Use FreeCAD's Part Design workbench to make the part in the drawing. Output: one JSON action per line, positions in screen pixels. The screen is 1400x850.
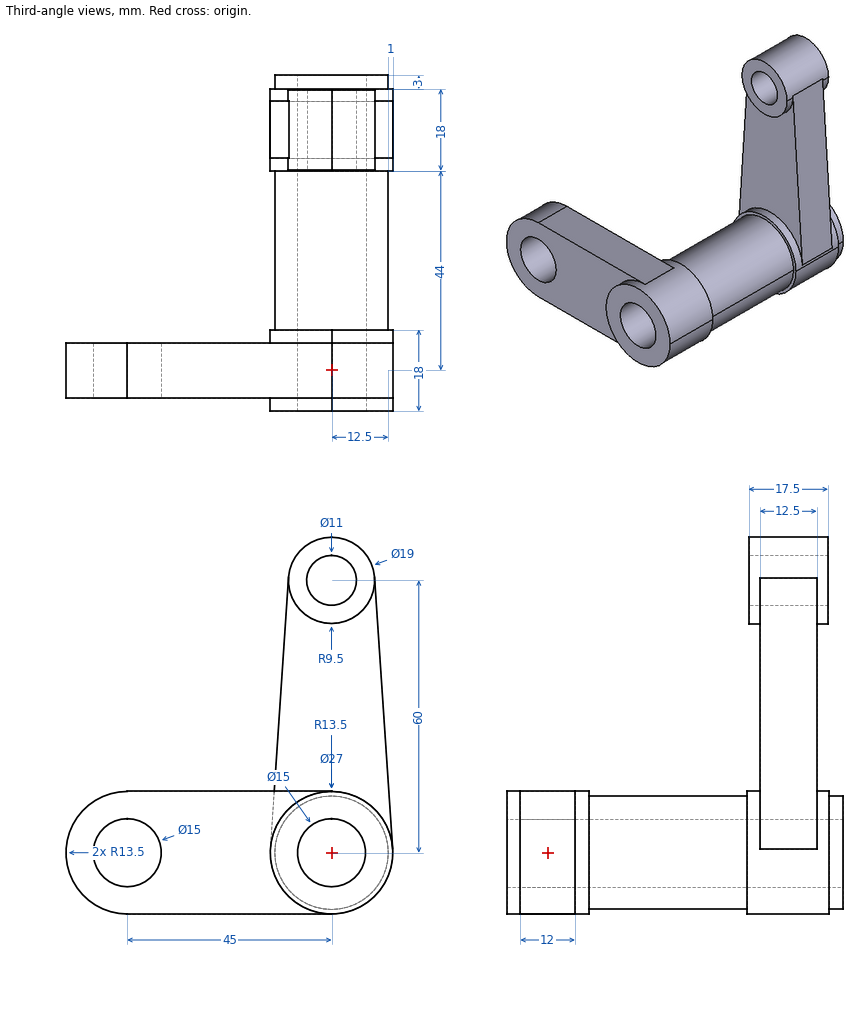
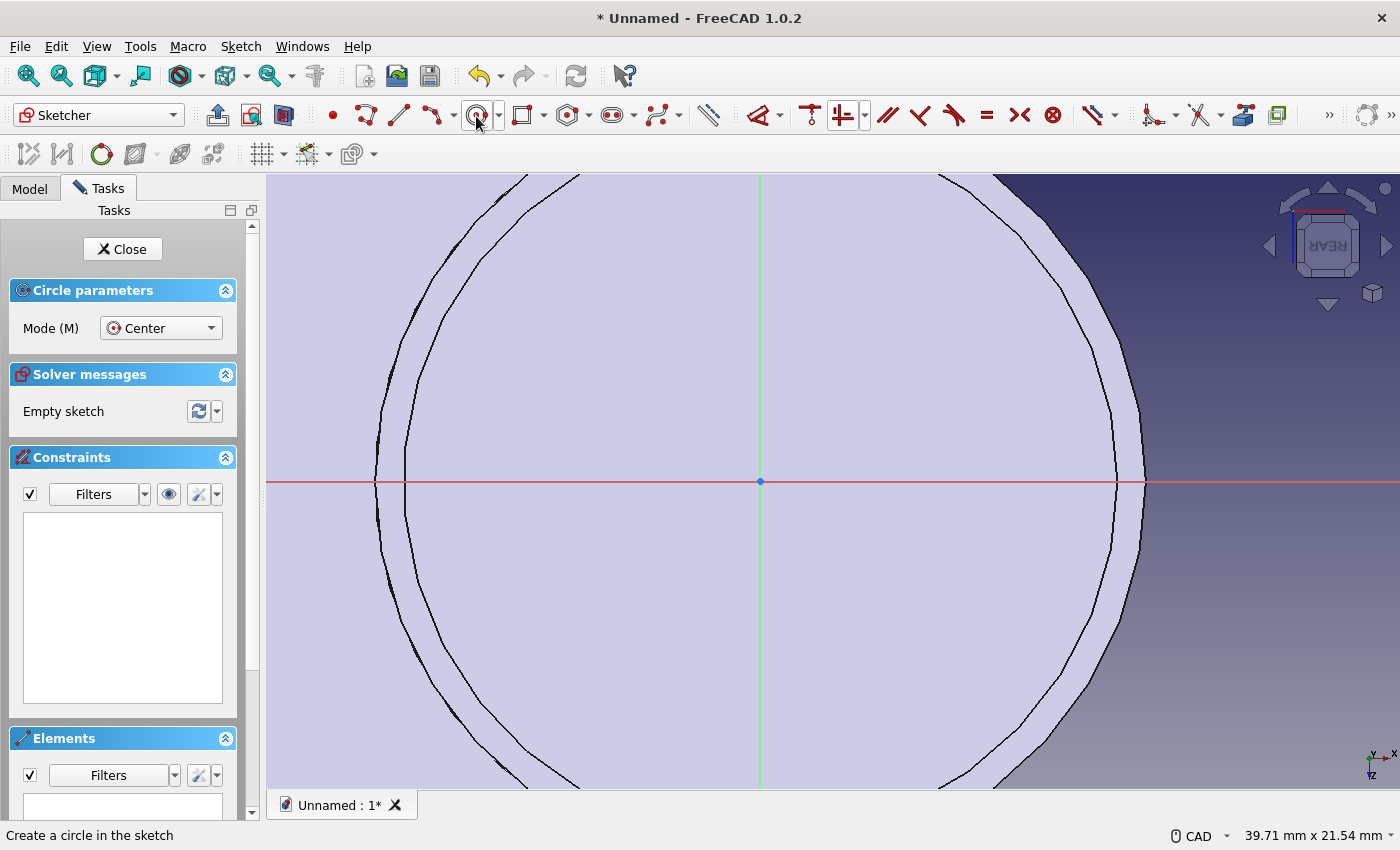
{"action": "left_click", "coordinate": [760, 481]}
{"action": "left_click", "coordinate": [912, 330]}
{"action": "key", "text": "Escape"}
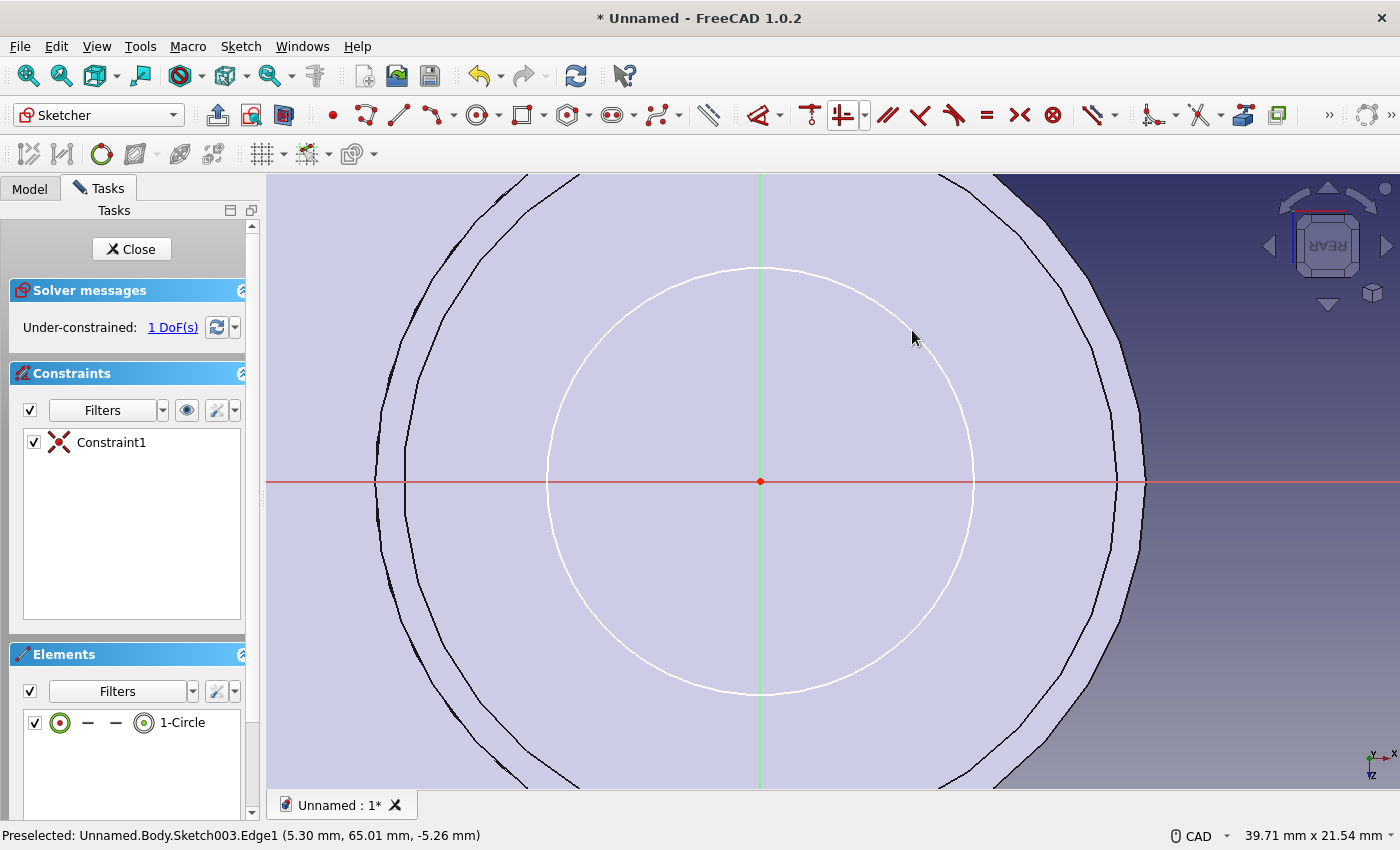
{"action": "left_click", "coordinate": [758, 116]}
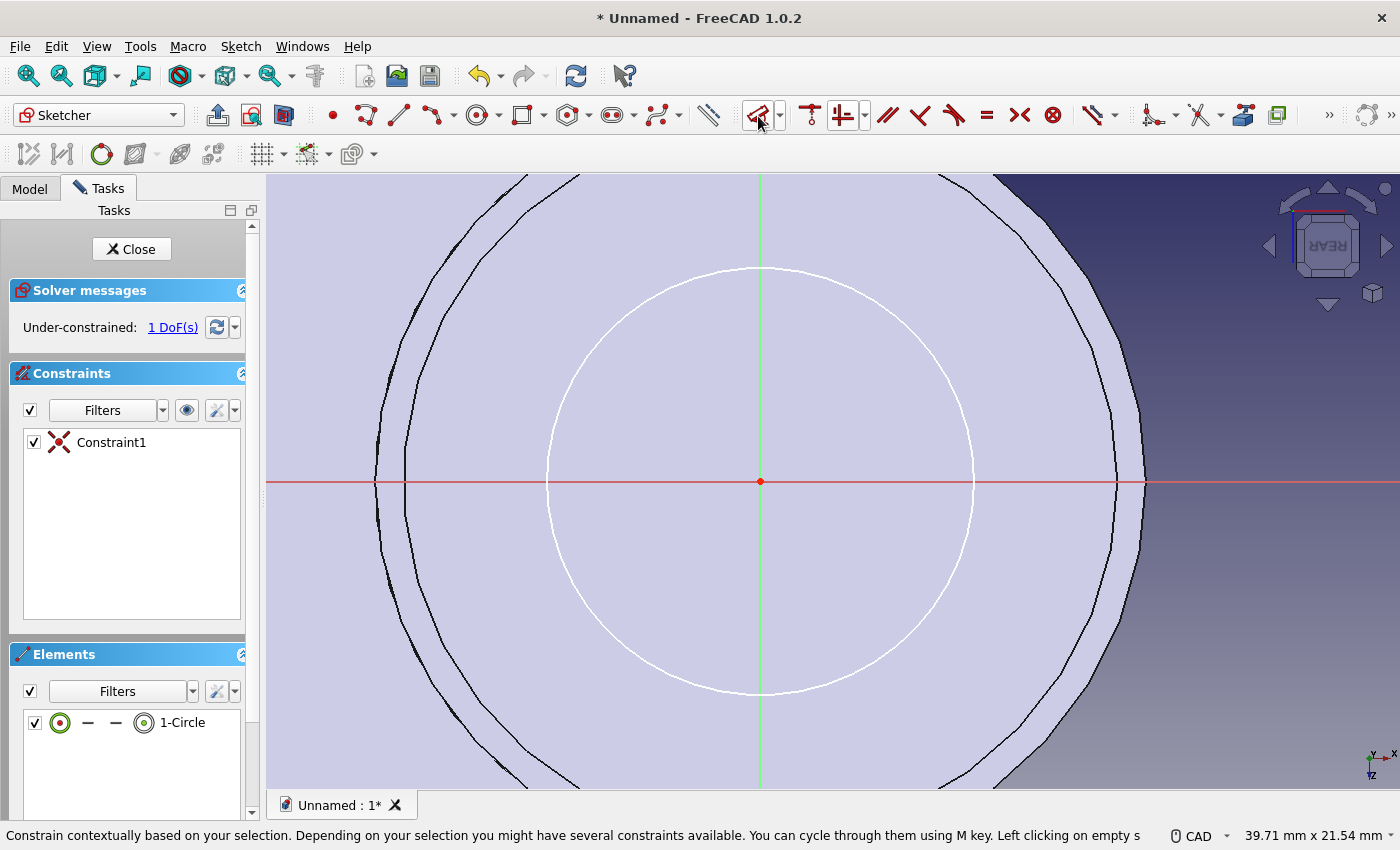
{"action": "left_click", "coordinate": [911, 330]}
{"action": "left_click", "coordinate": [934, 307]}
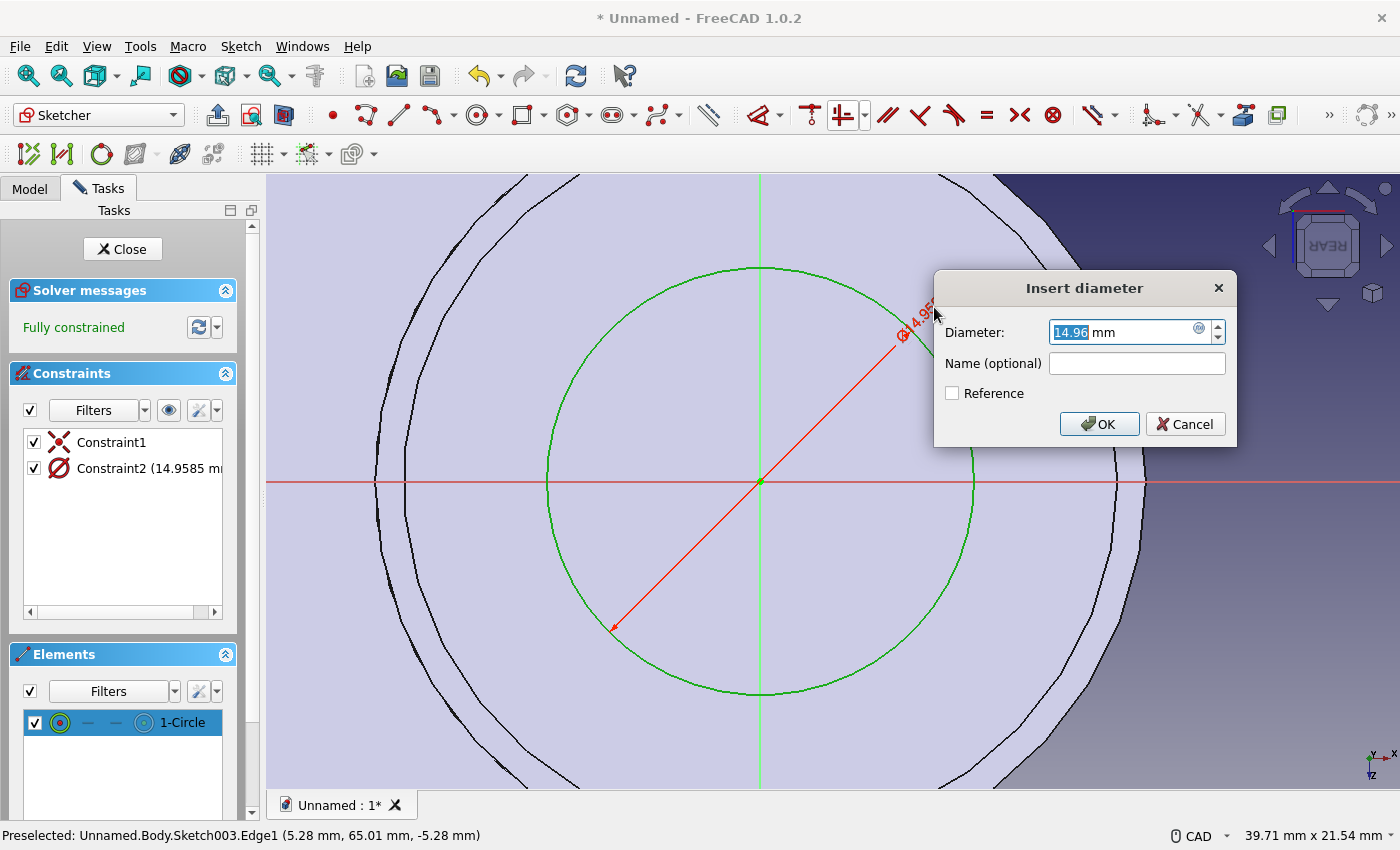
{"action": "type", "text": "15"}
{"action": "key", "text": "Return"}
{"action": "key", "text": "Escape"}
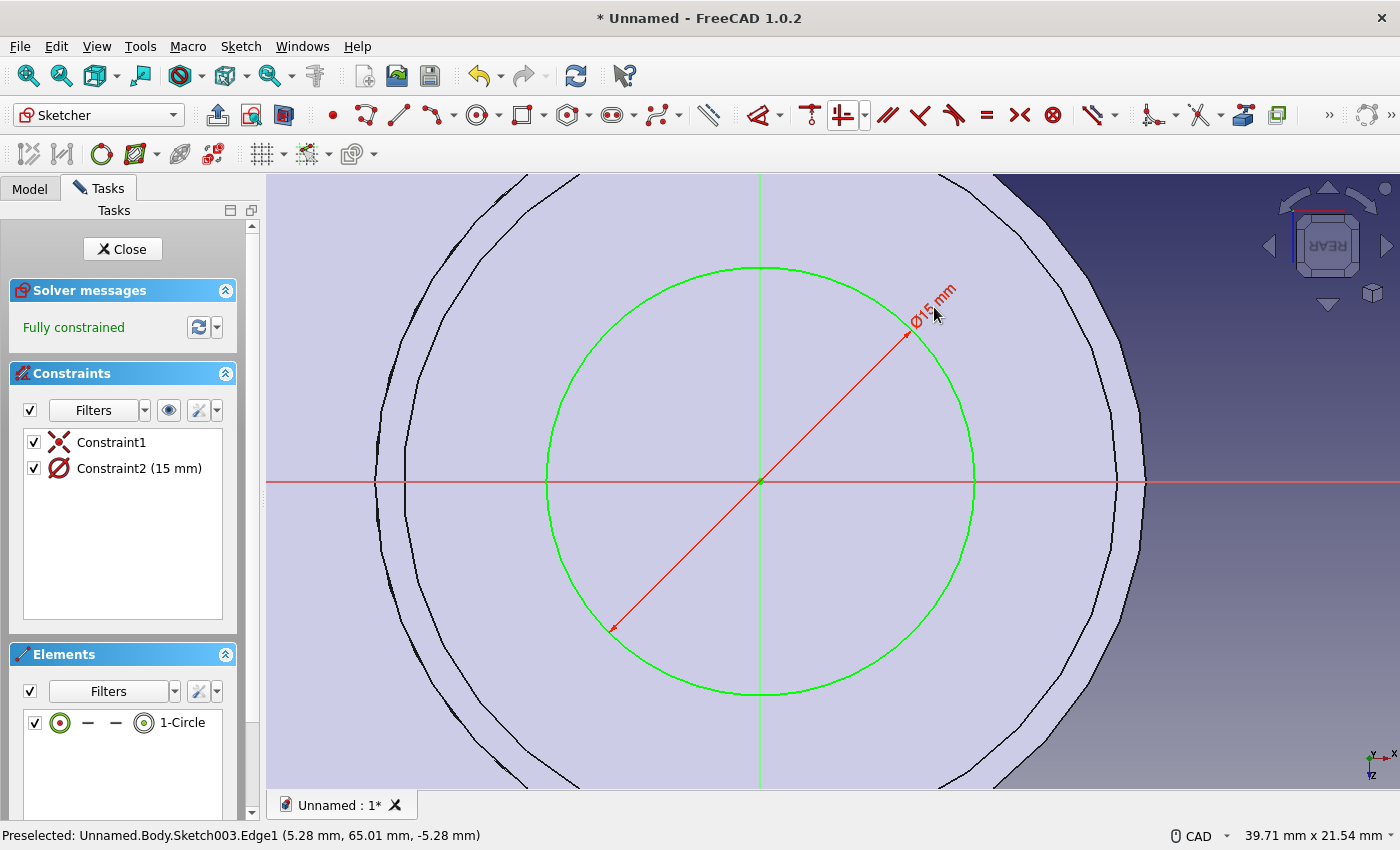
{"action": "left_click", "coordinate": [123, 249]}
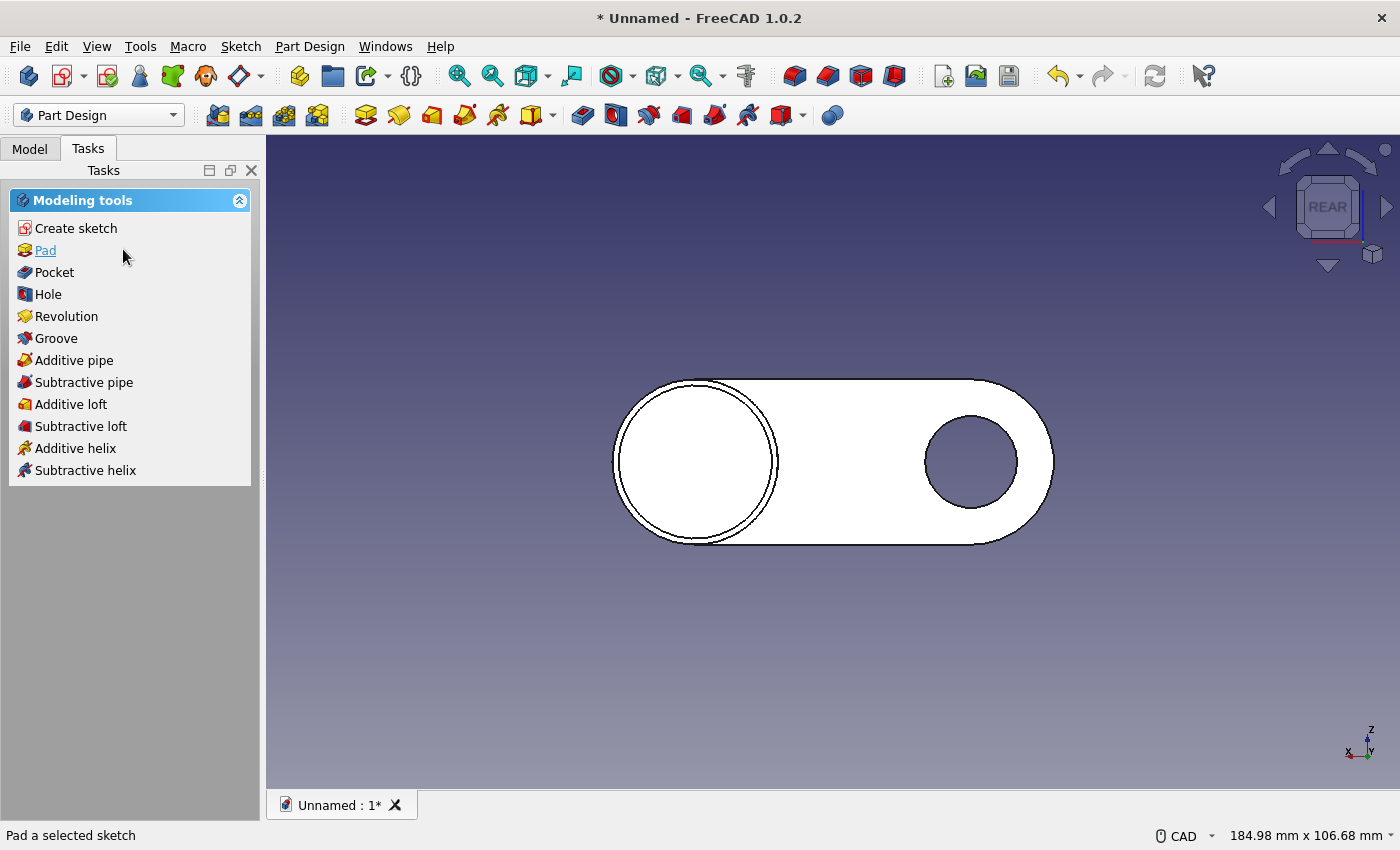
{"action": "left_click", "coordinate": [583, 116]}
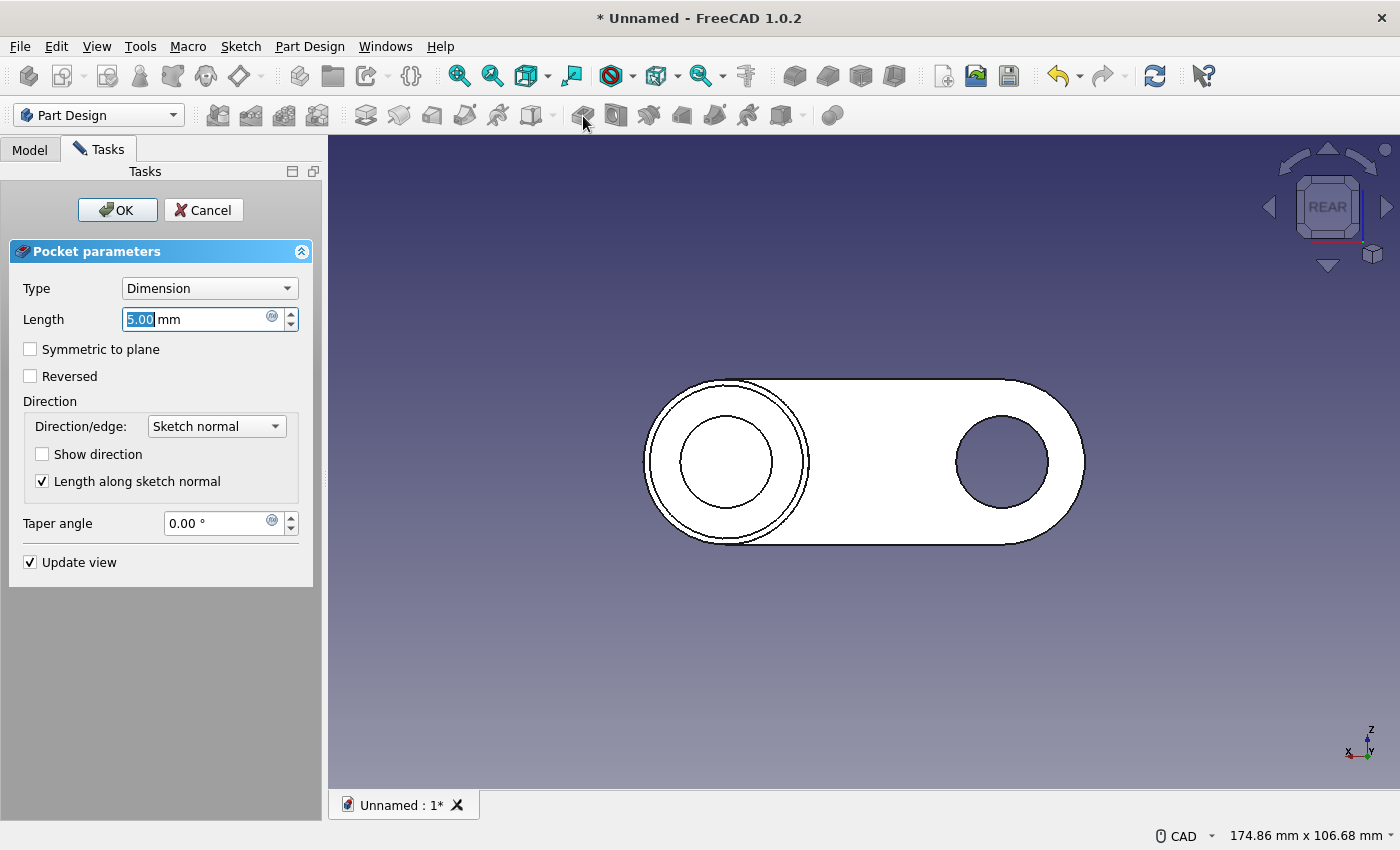
{"action": "left_click", "coordinate": [210, 288]}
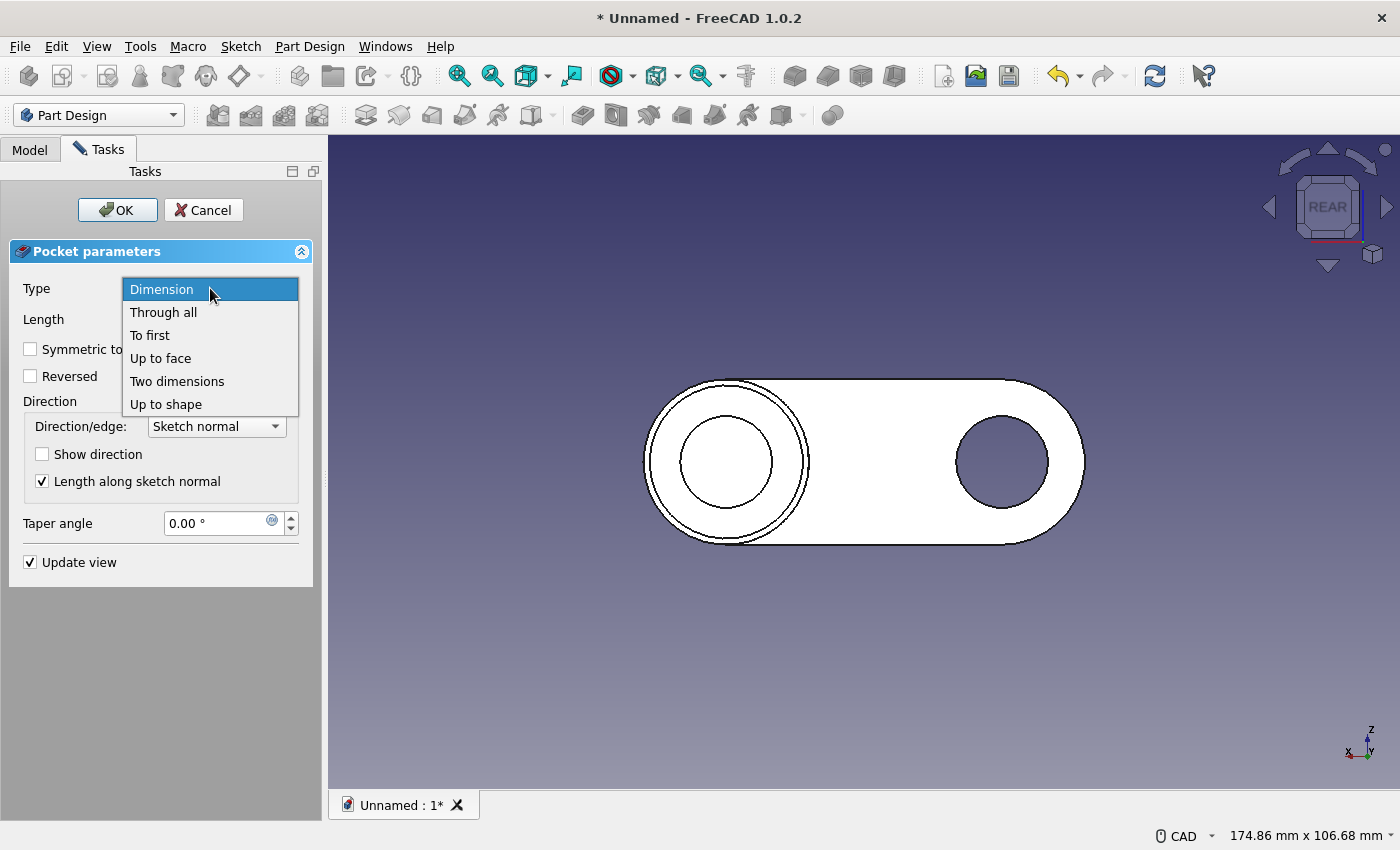
{"action": "left_click", "coordinate": [208, 312]}